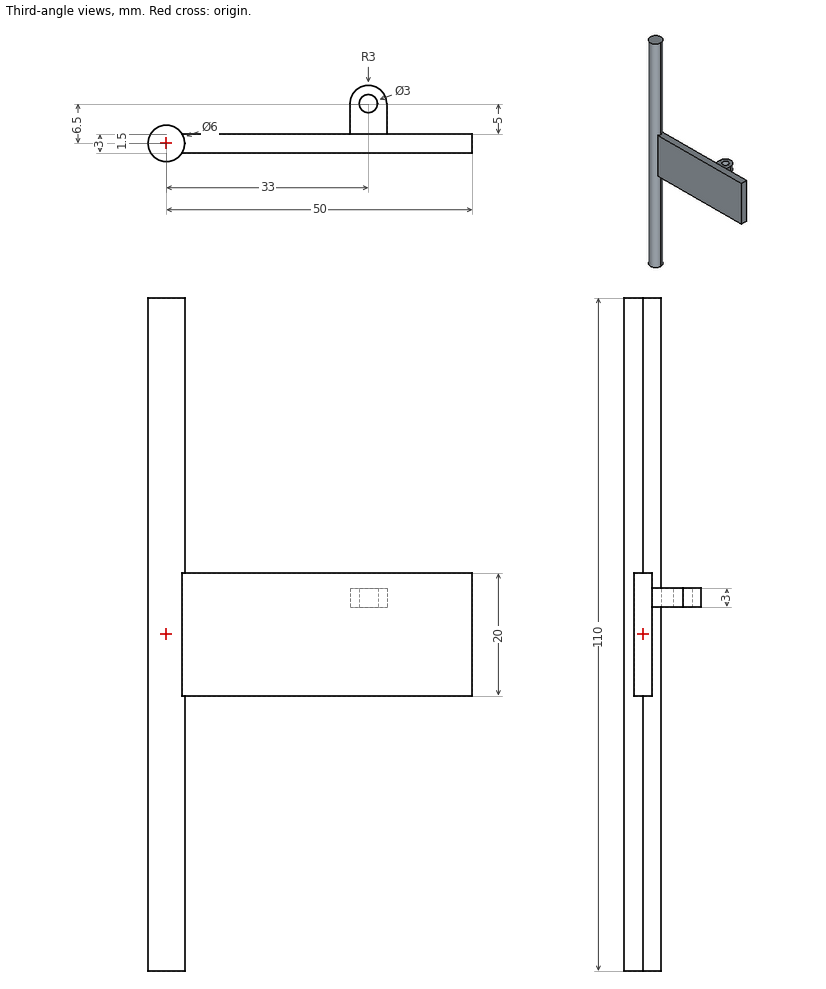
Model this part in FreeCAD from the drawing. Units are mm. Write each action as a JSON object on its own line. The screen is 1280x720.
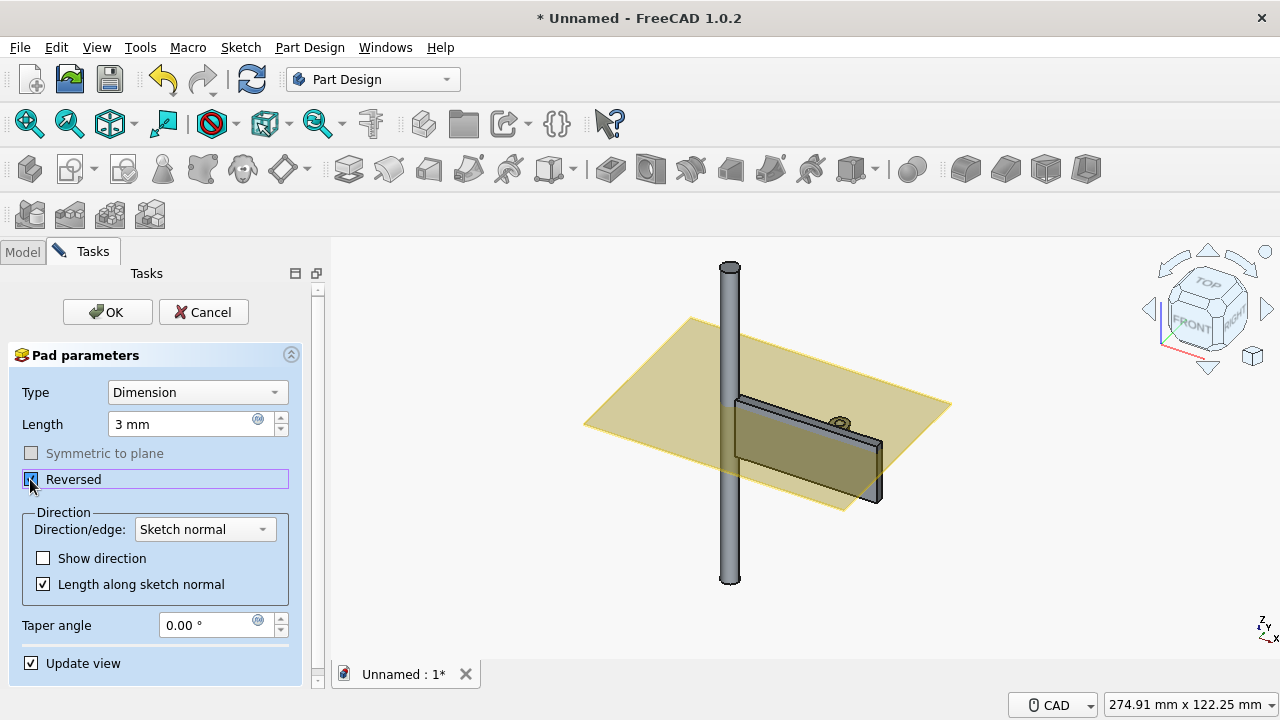
{"action": "left_click", "coordinate": [108, 312]}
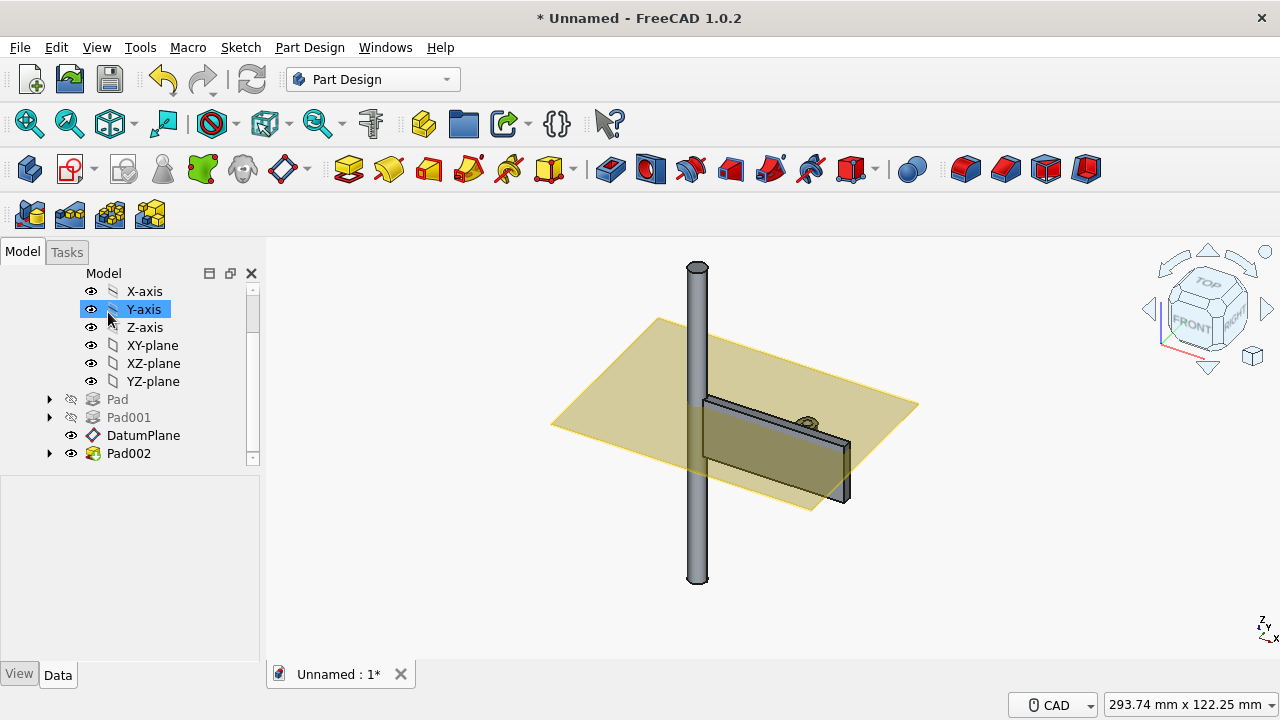
{"action": "left_click", "coordinate": [116, 435]}
{"action": "key", "text": "space"}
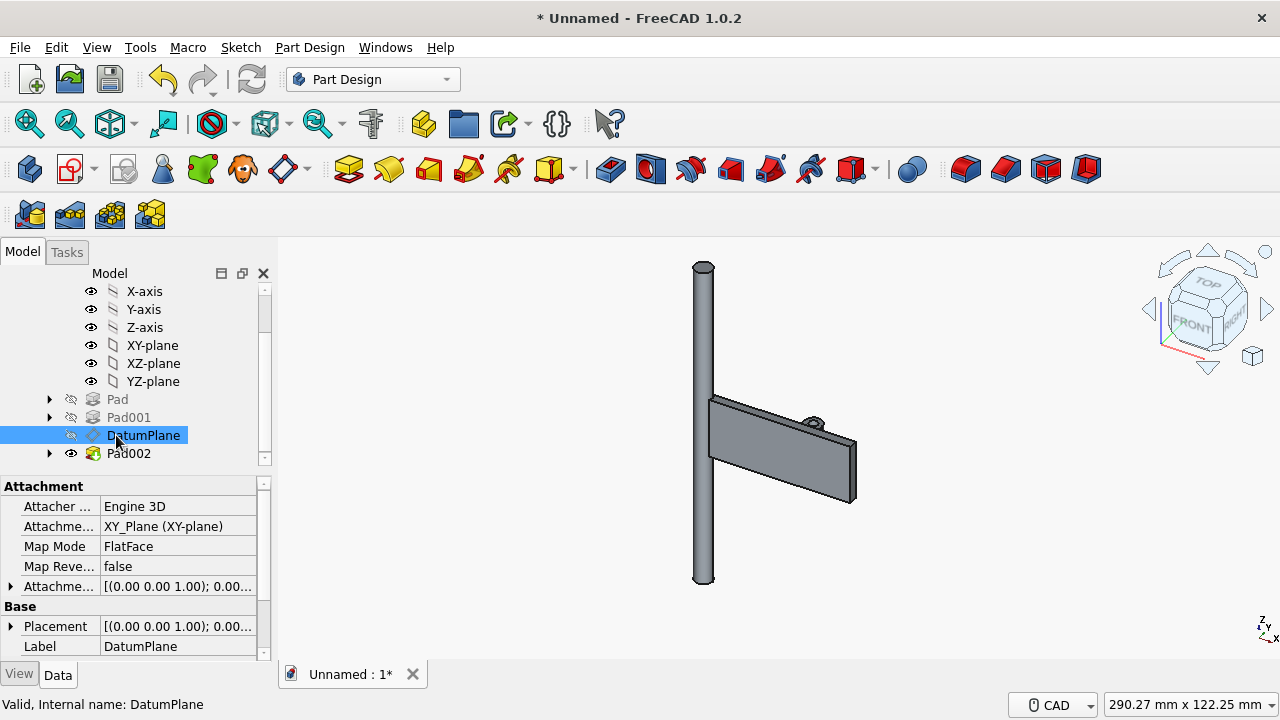
{"action": "key", "text": "0"}